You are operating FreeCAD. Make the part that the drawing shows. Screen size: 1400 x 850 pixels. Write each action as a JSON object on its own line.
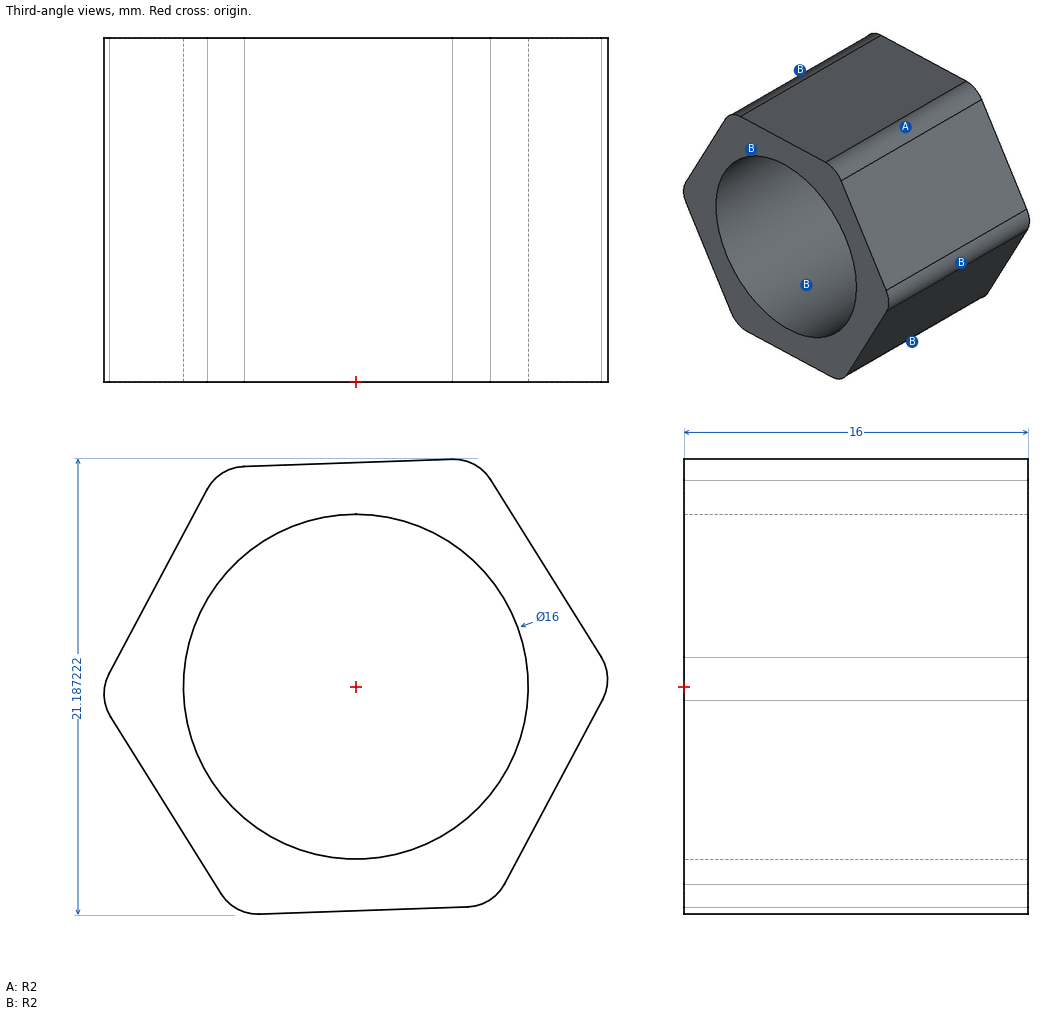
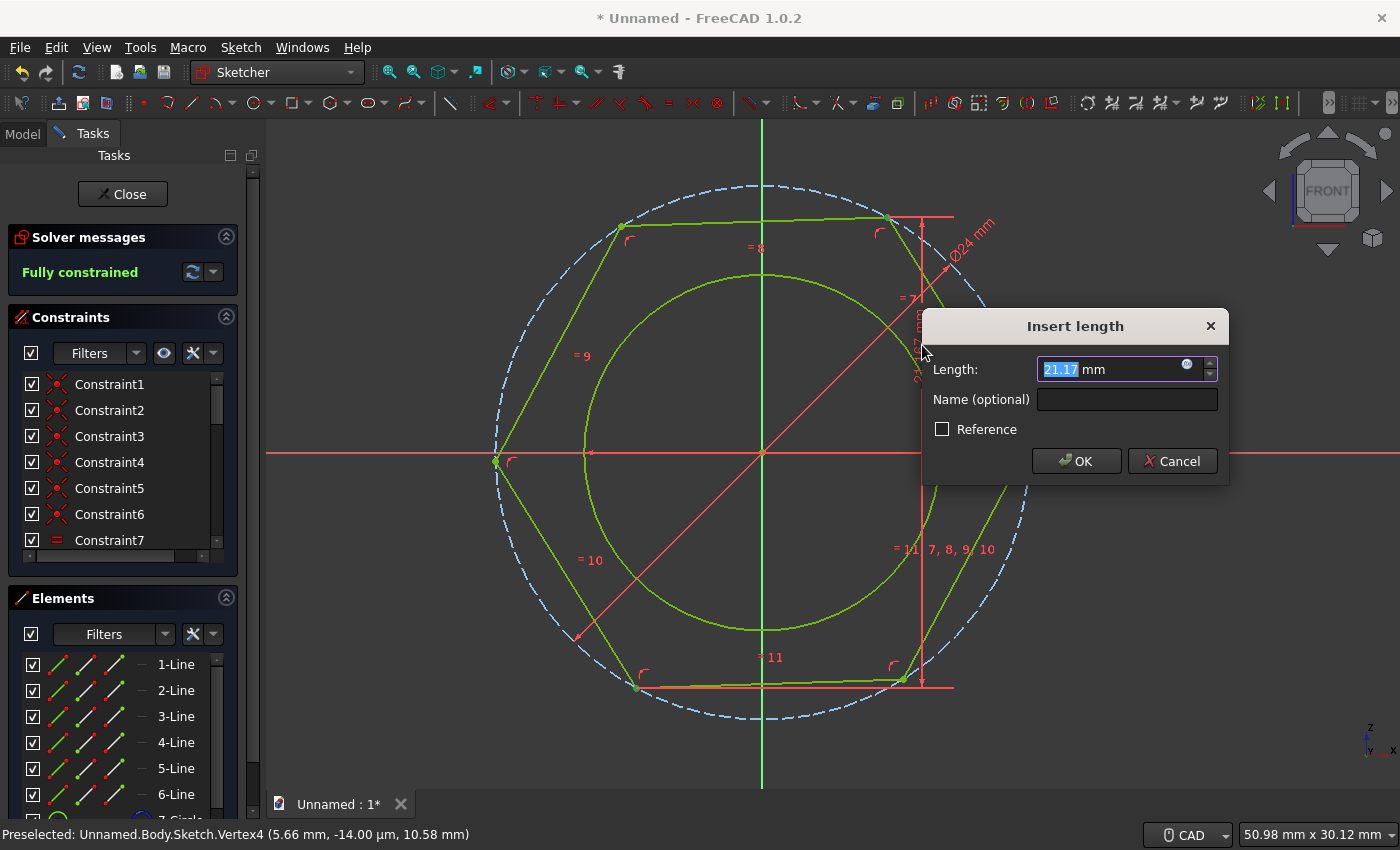
{"action": "type", "text": "21.187222"}
{"action": "key", "text": "Return"}
{"action": "key", "text": "Escape"}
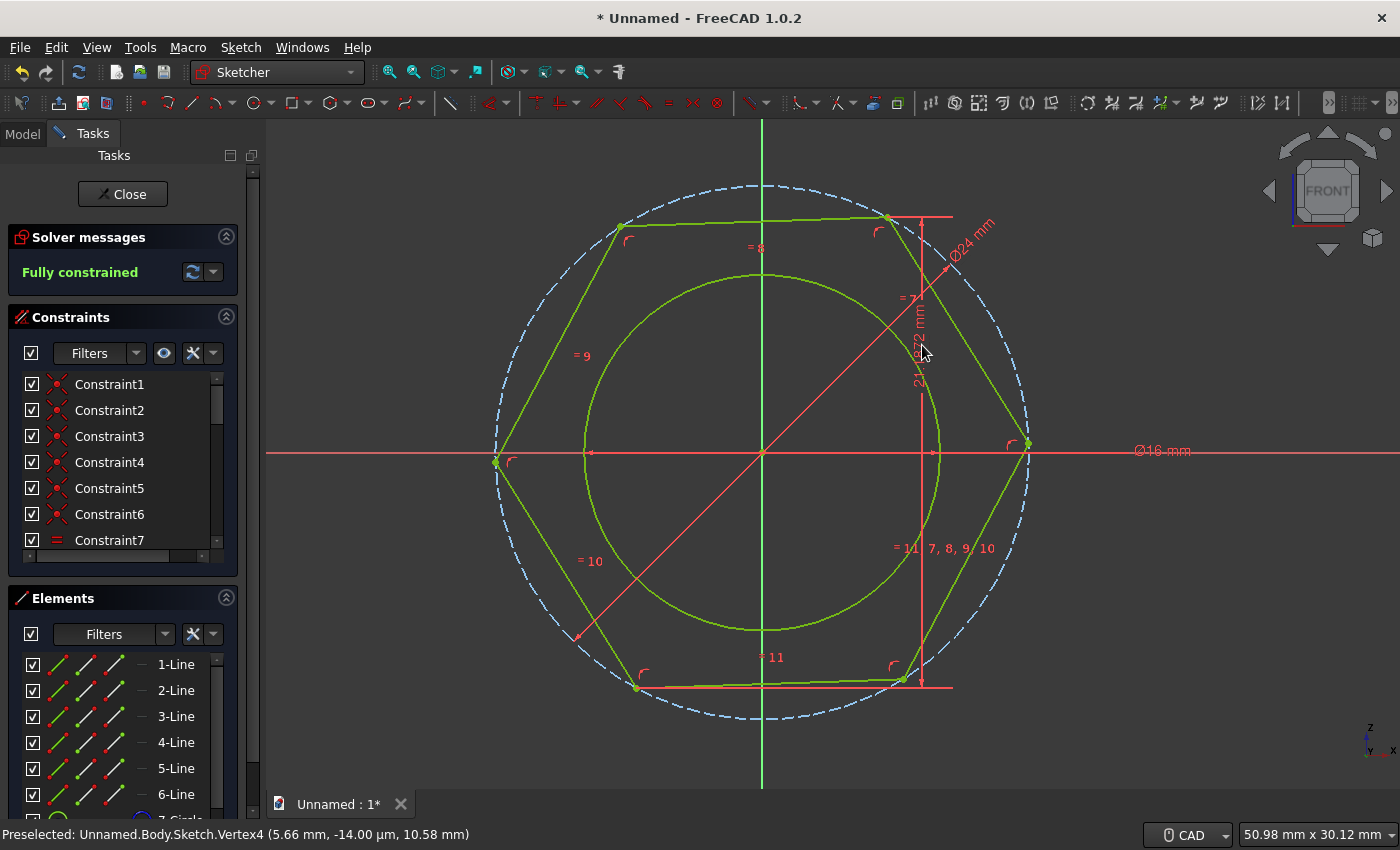
{"action": "left_click", "coordinate": [123, 194]}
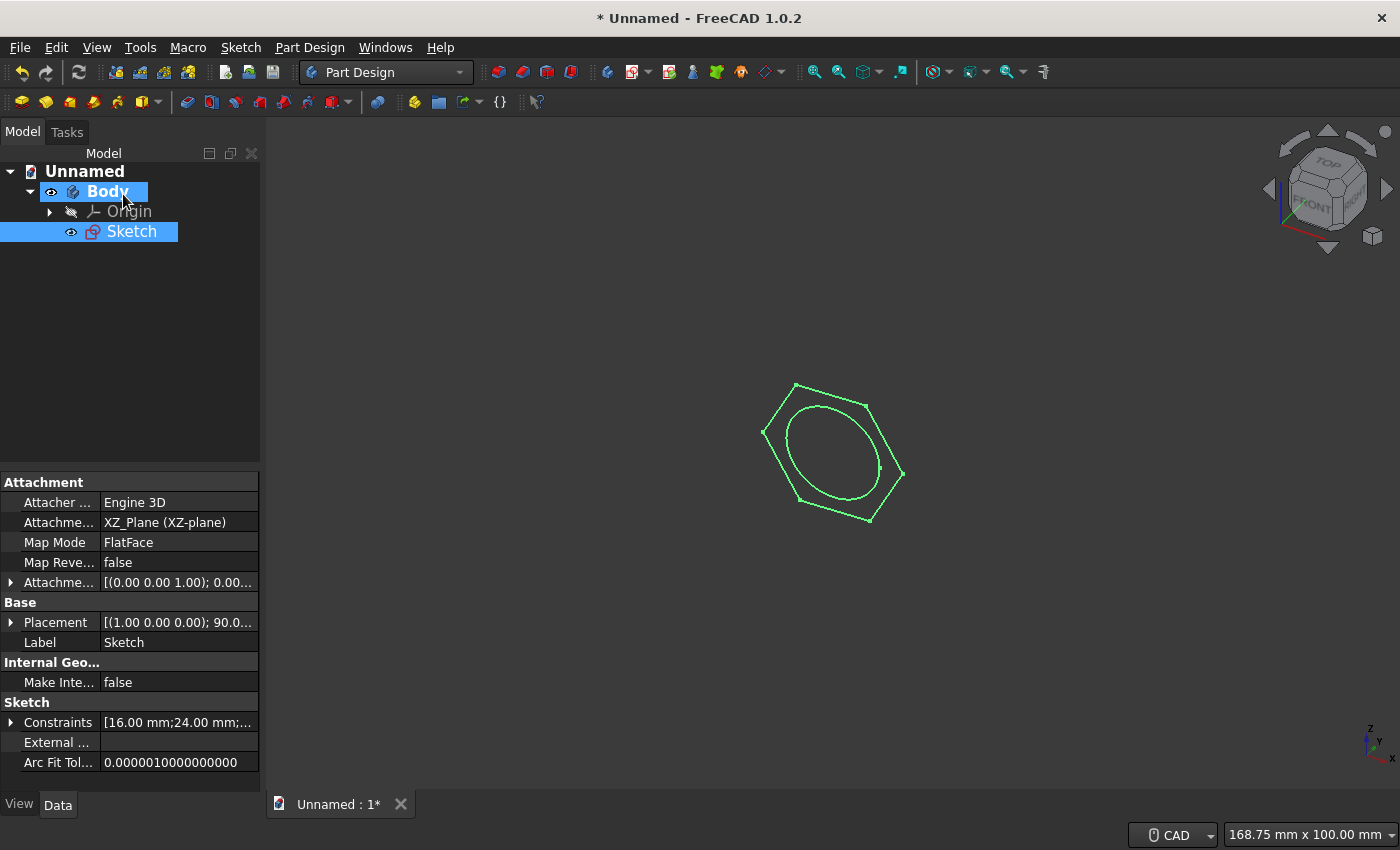
{"action": "left_click", "coordinate": [22, 102]}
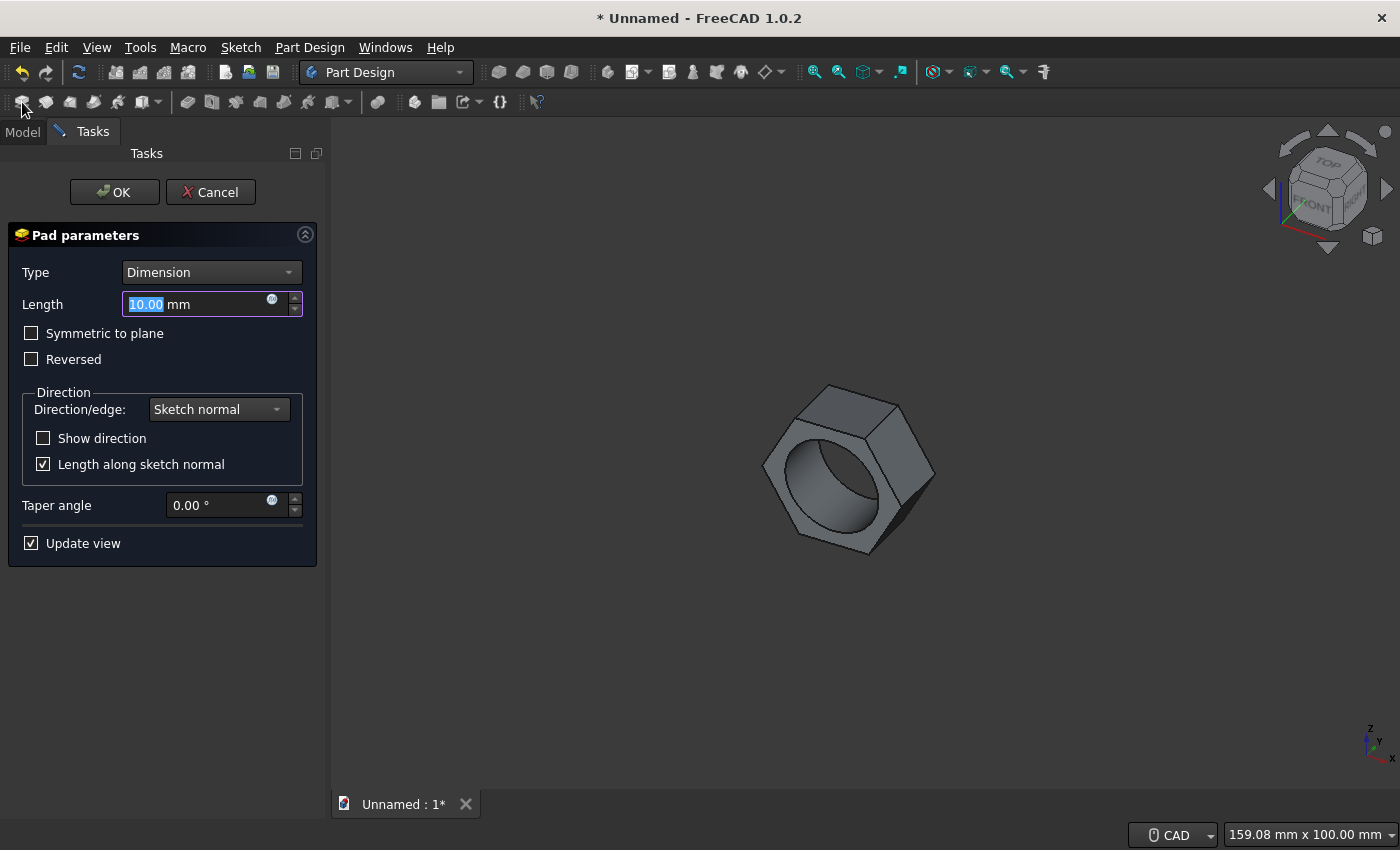
{"action": "type", "text": "16"}
{"action": "key", "text": "Tab"}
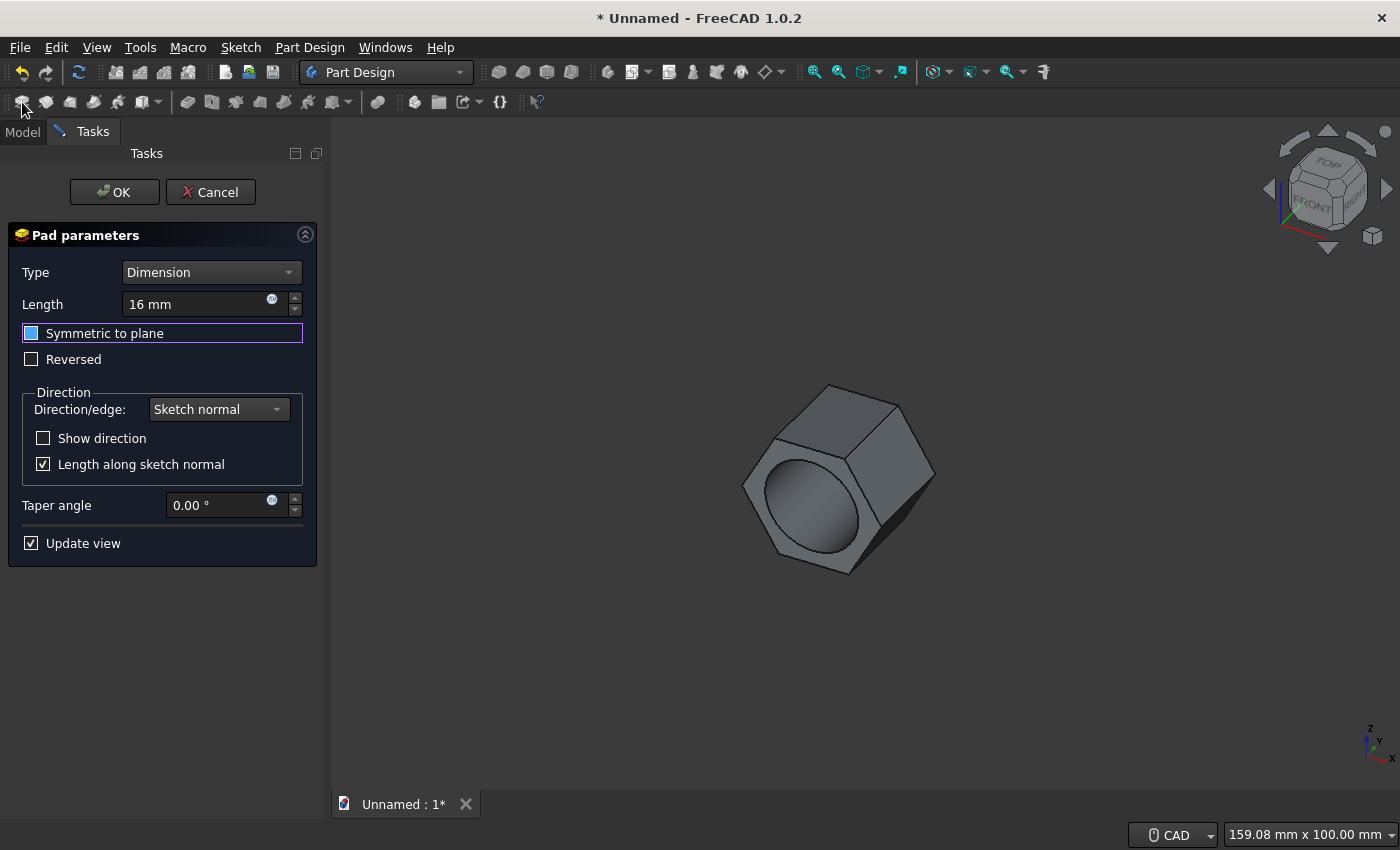
{"action": "left_click", "coordinate": [30, 359]}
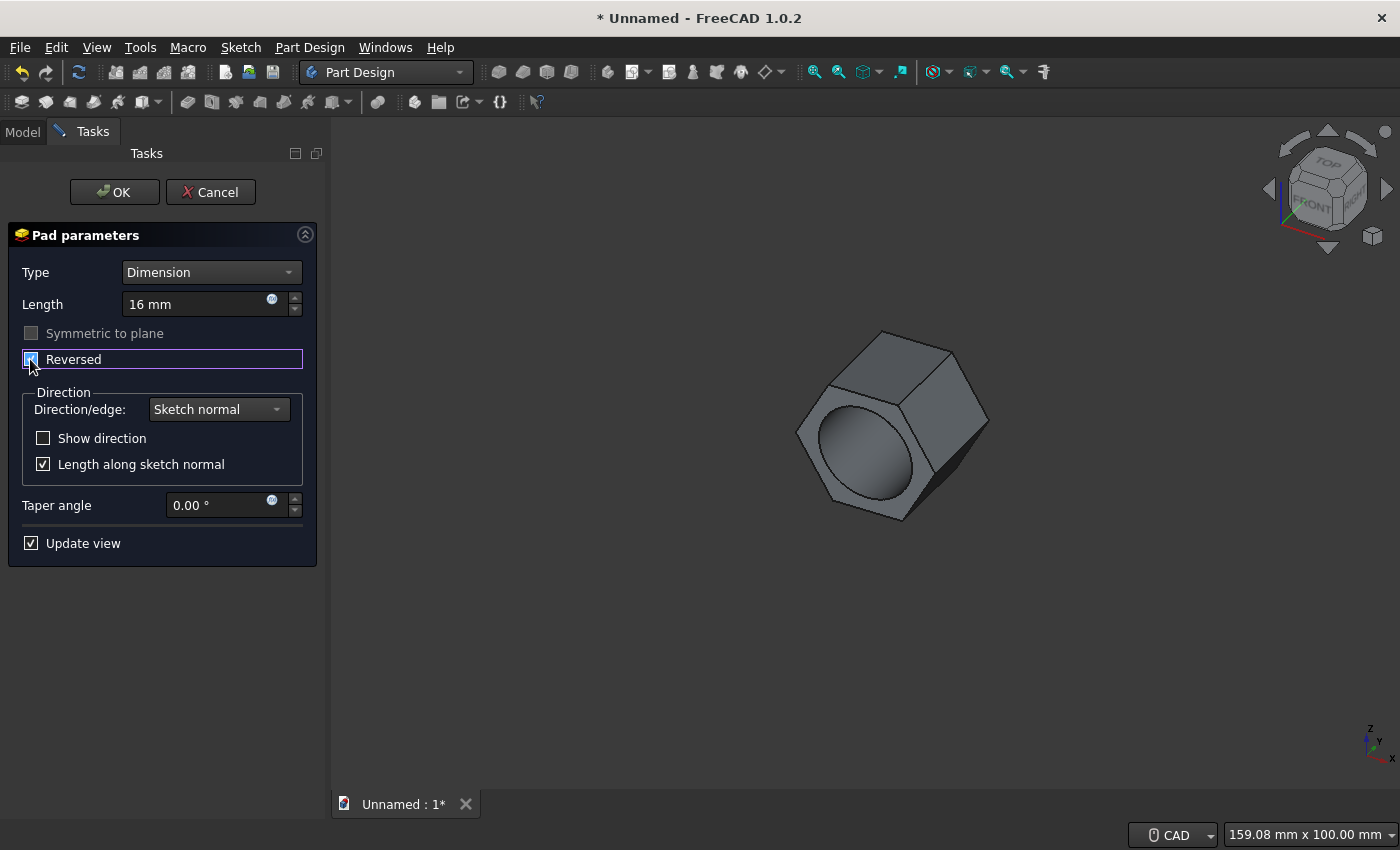
{"action": "left_click", "coordinate": [115, 192]}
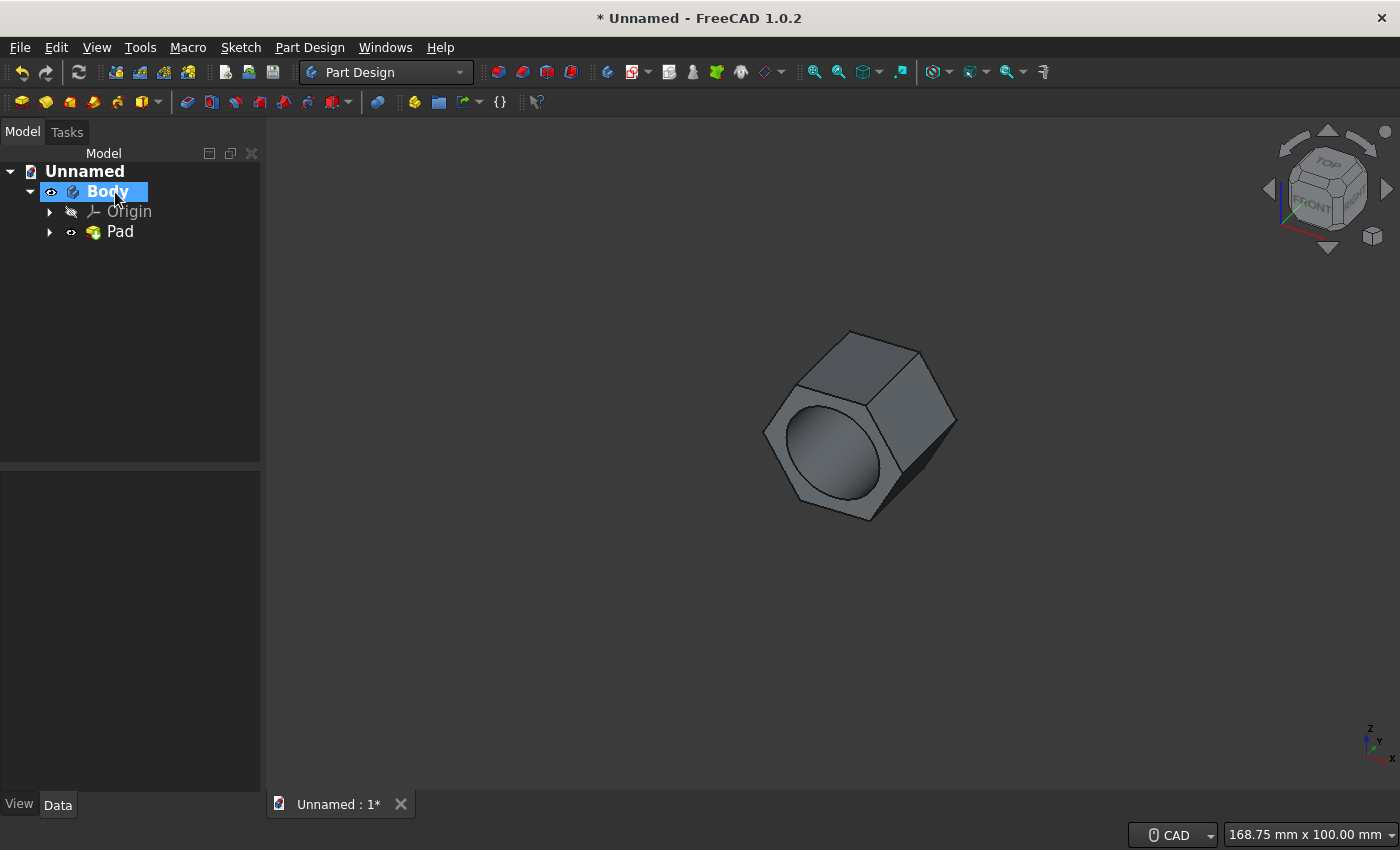
{"action": "left_click", "coordinate": [816, 72]}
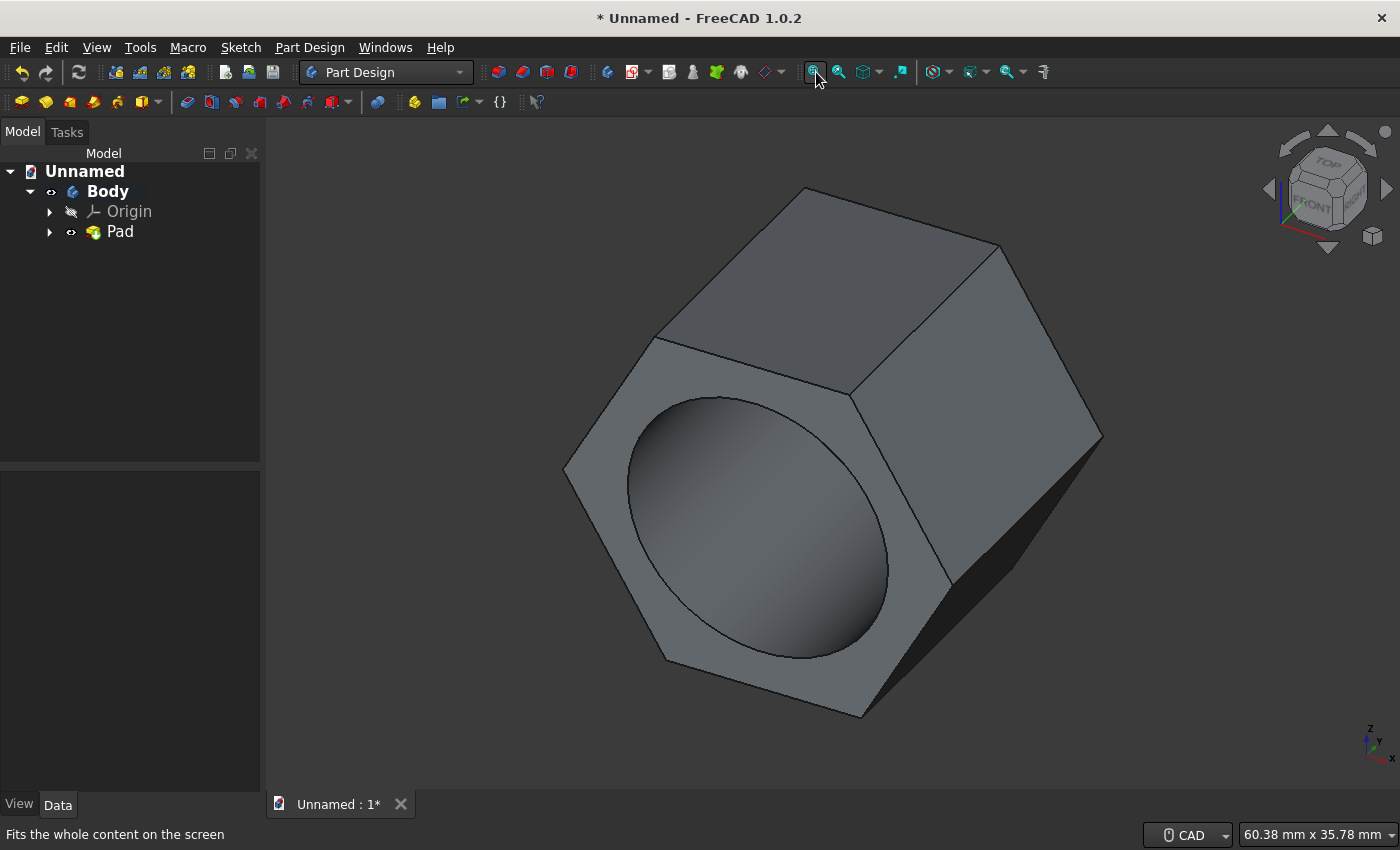
{"action": "left_click", "coordinate": [925, 319]}